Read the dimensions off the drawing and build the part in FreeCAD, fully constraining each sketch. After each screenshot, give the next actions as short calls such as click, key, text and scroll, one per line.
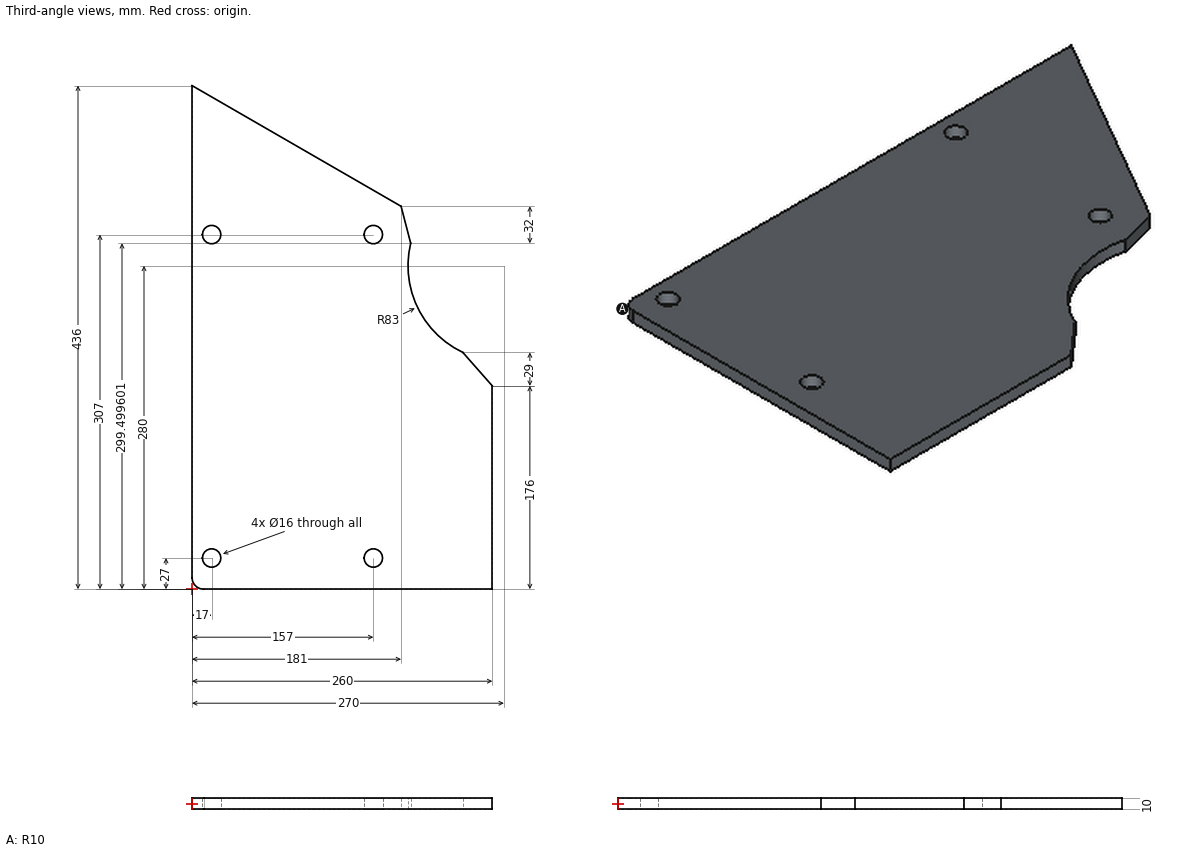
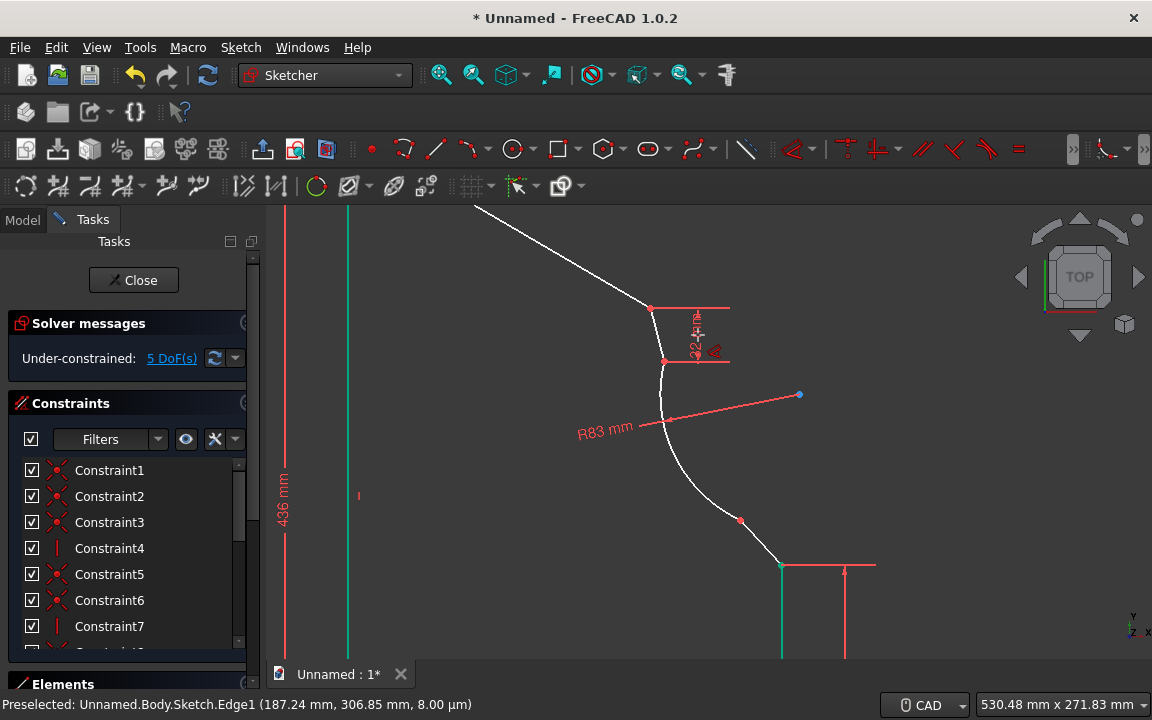
click(769, 552)
click(816, 543)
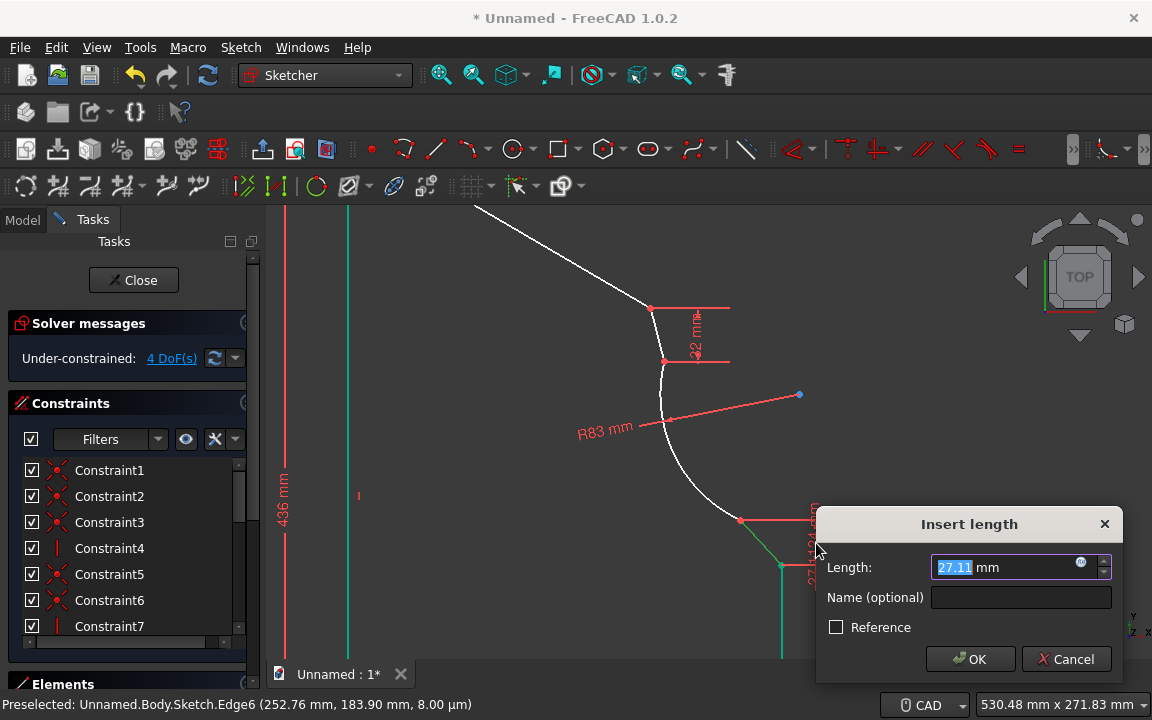
text(29)
key(Return)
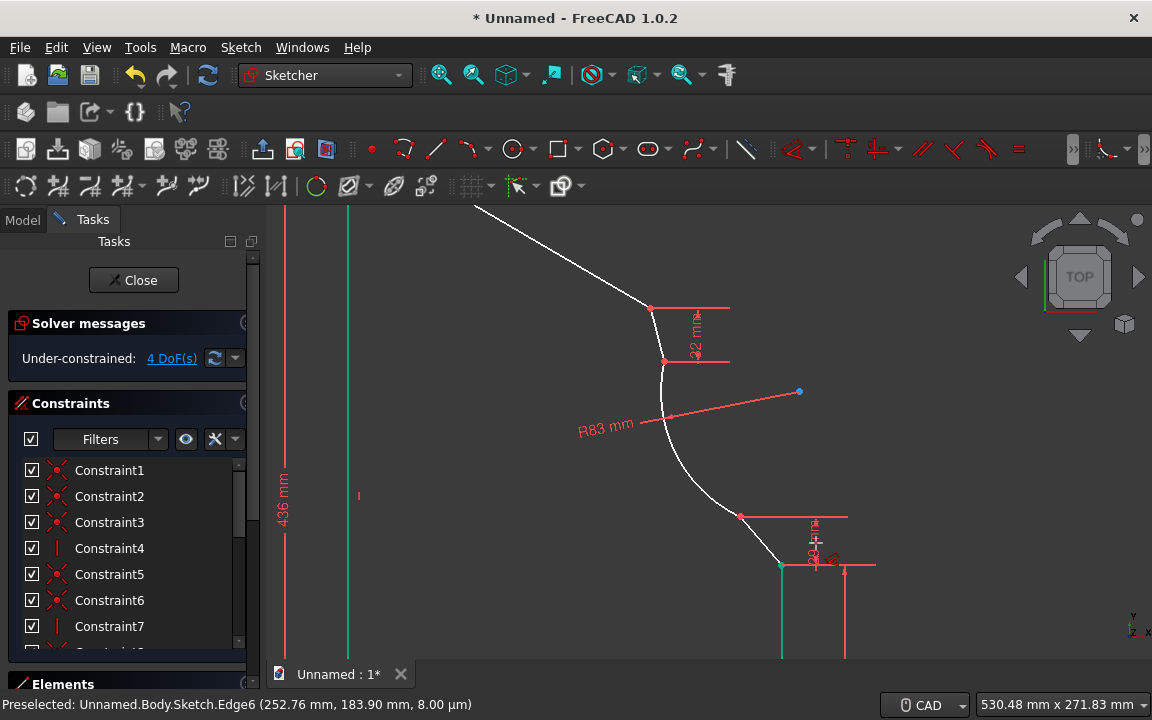
click(651, 308)
click(499, 274)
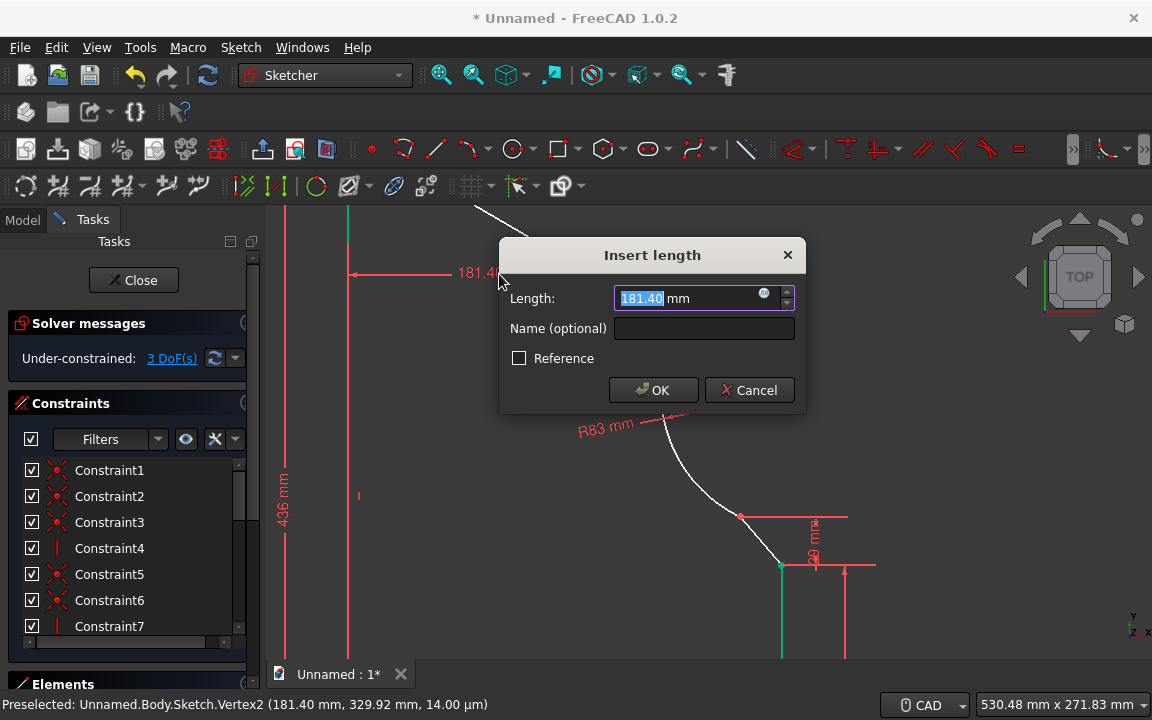
text(181)
key(Return)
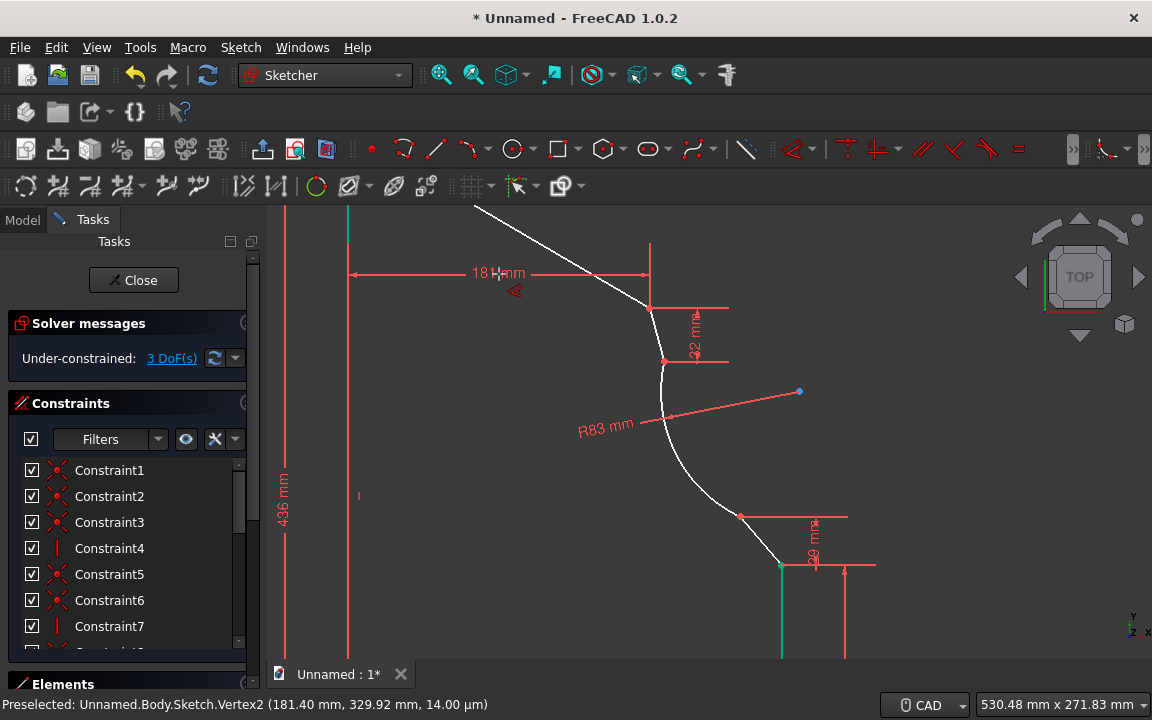
click(800, 392)
click(574, 358)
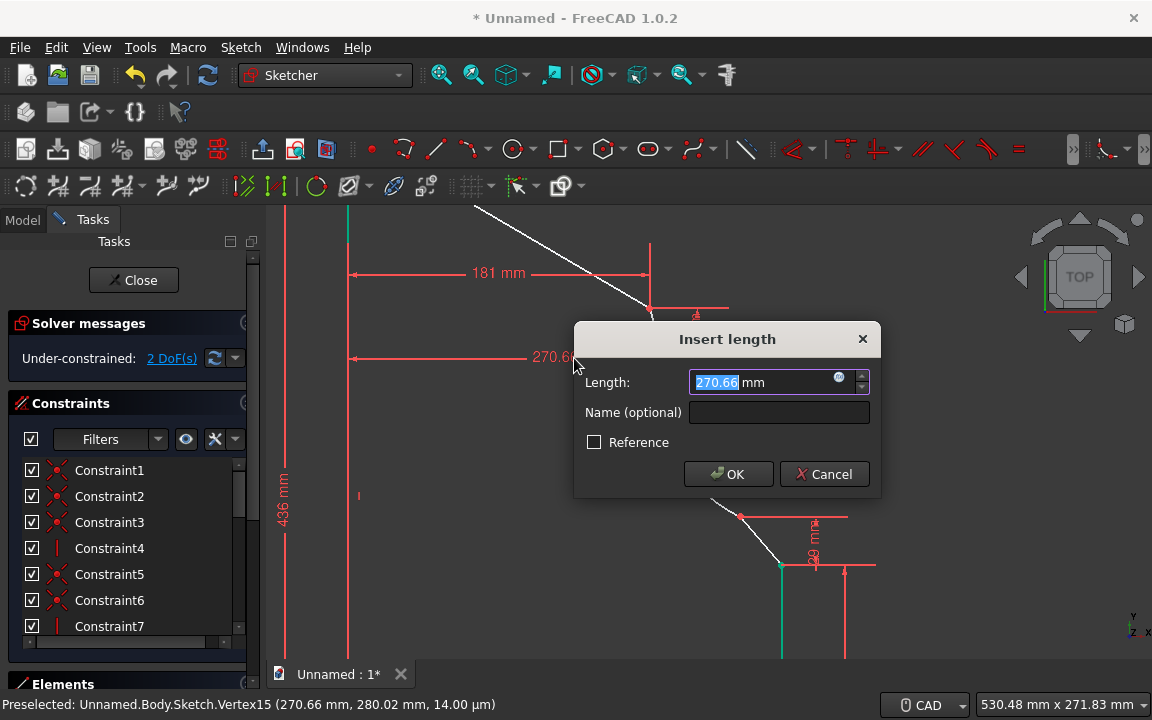
text(270)
key(Return)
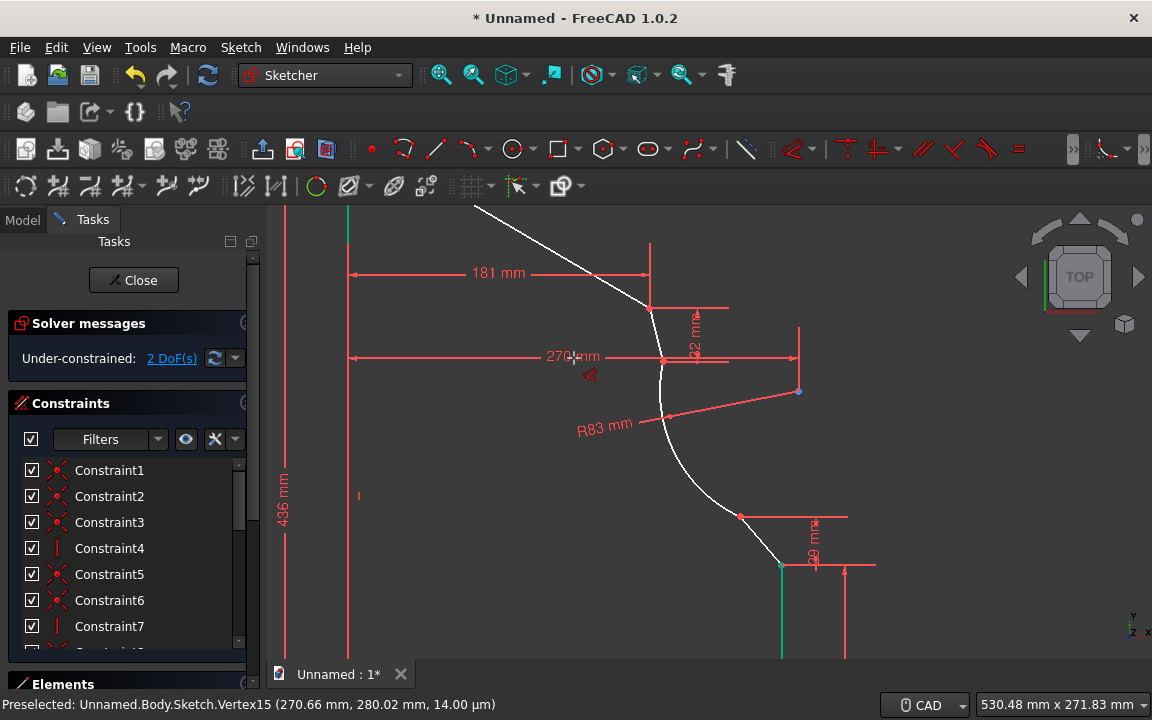
click(799, 391)
click(833, 511)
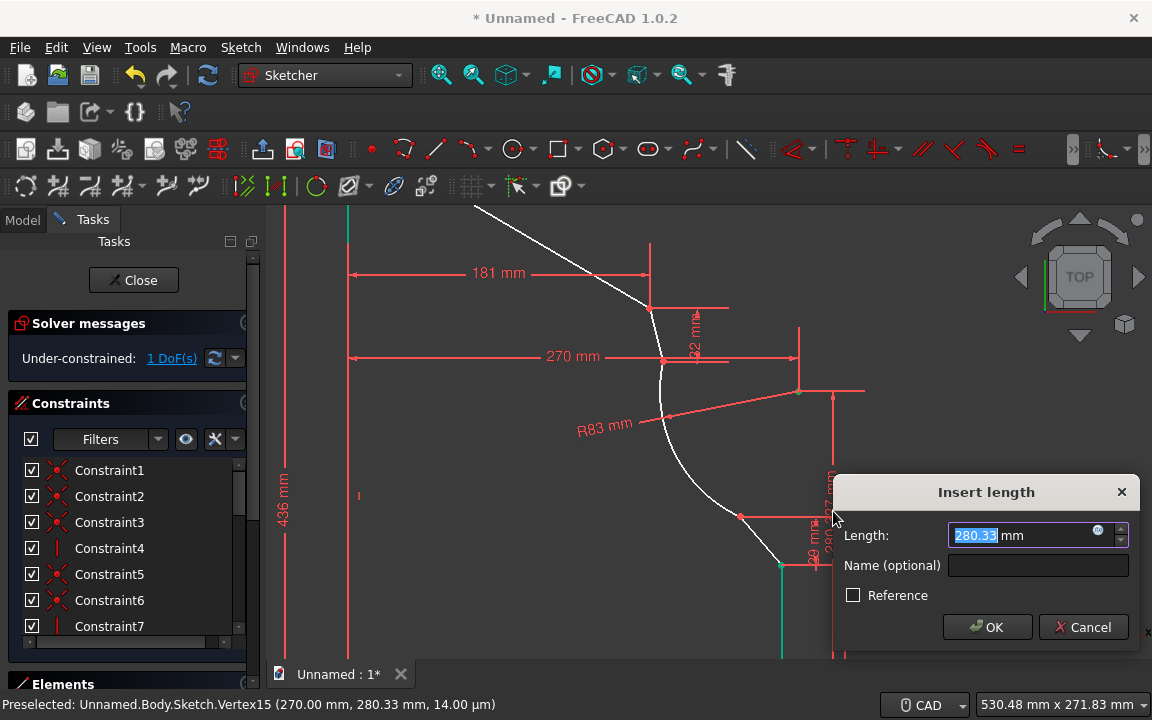
text(280)
key(Return)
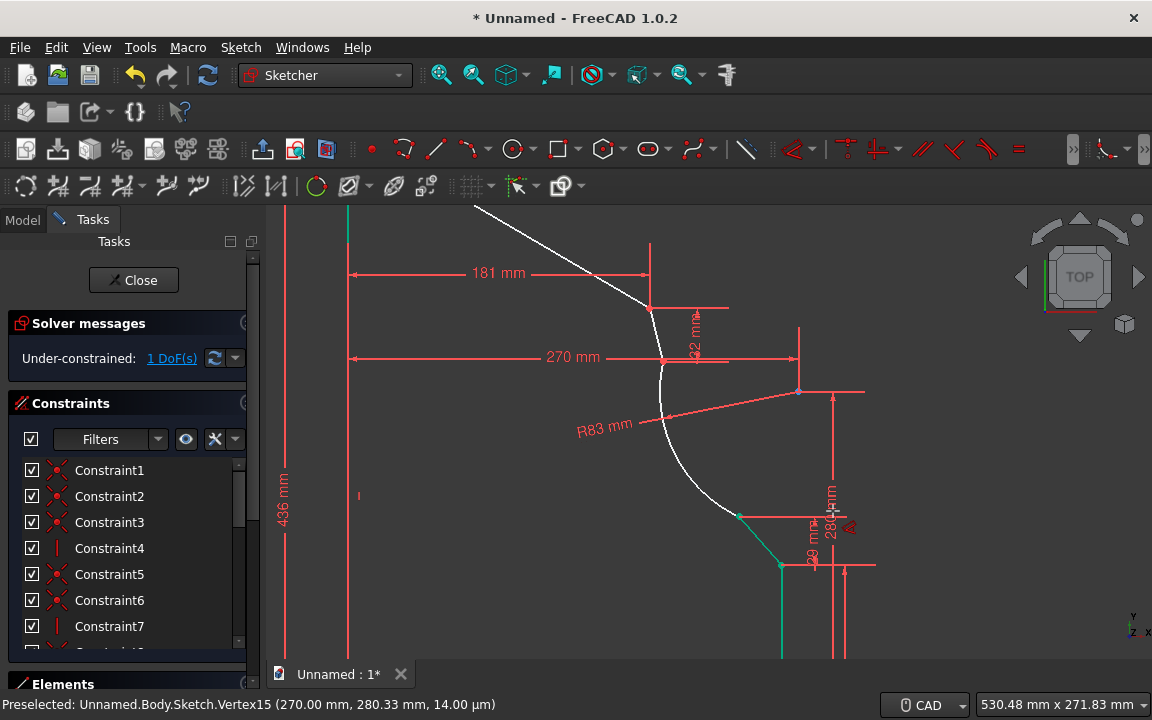
click(663, 362)
click(314, 434)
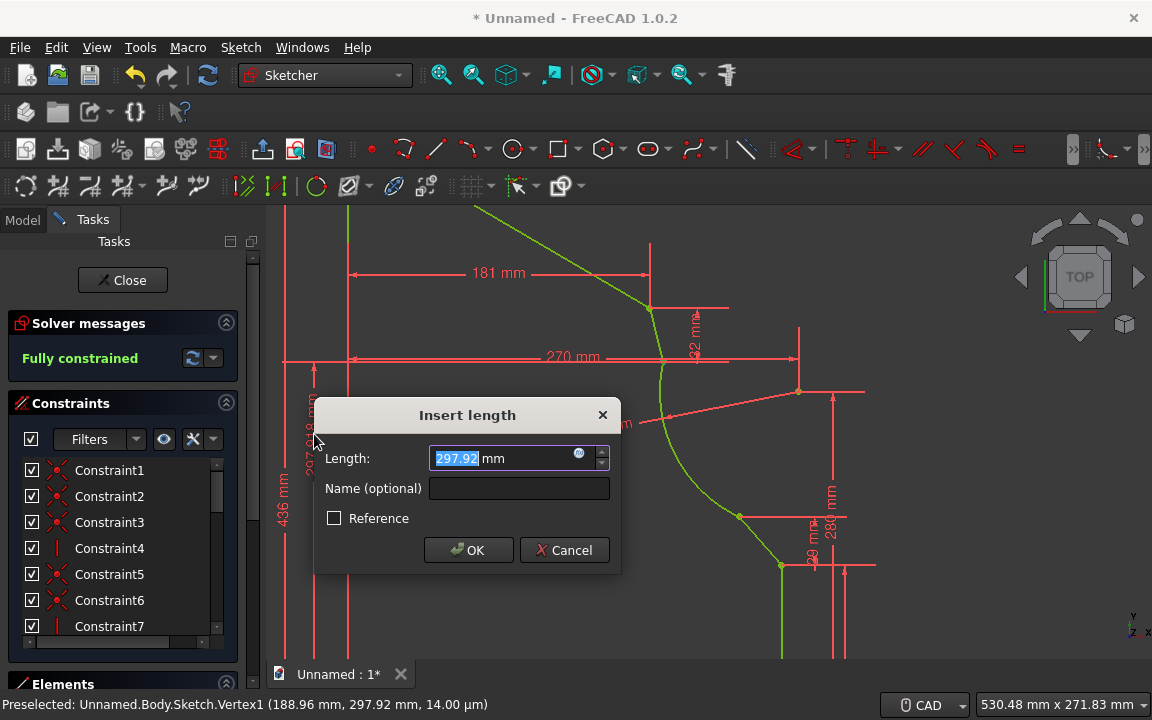
text(299.499601)
key(Return)
key(Escape)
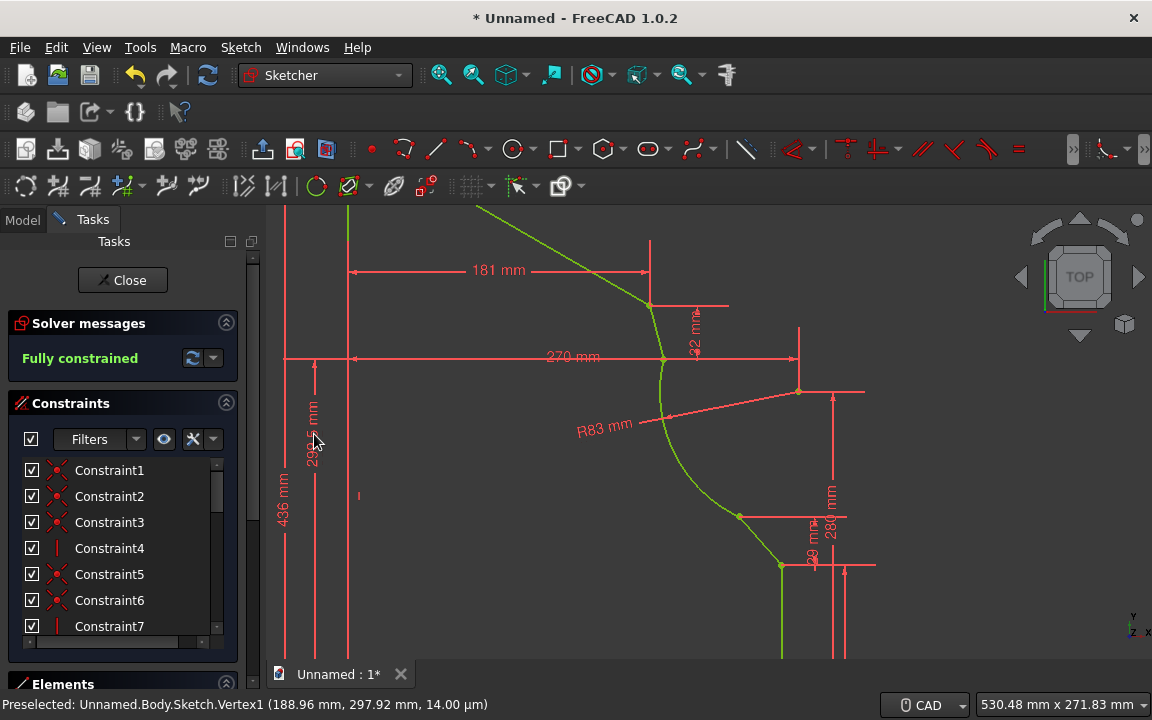
click(123, 280)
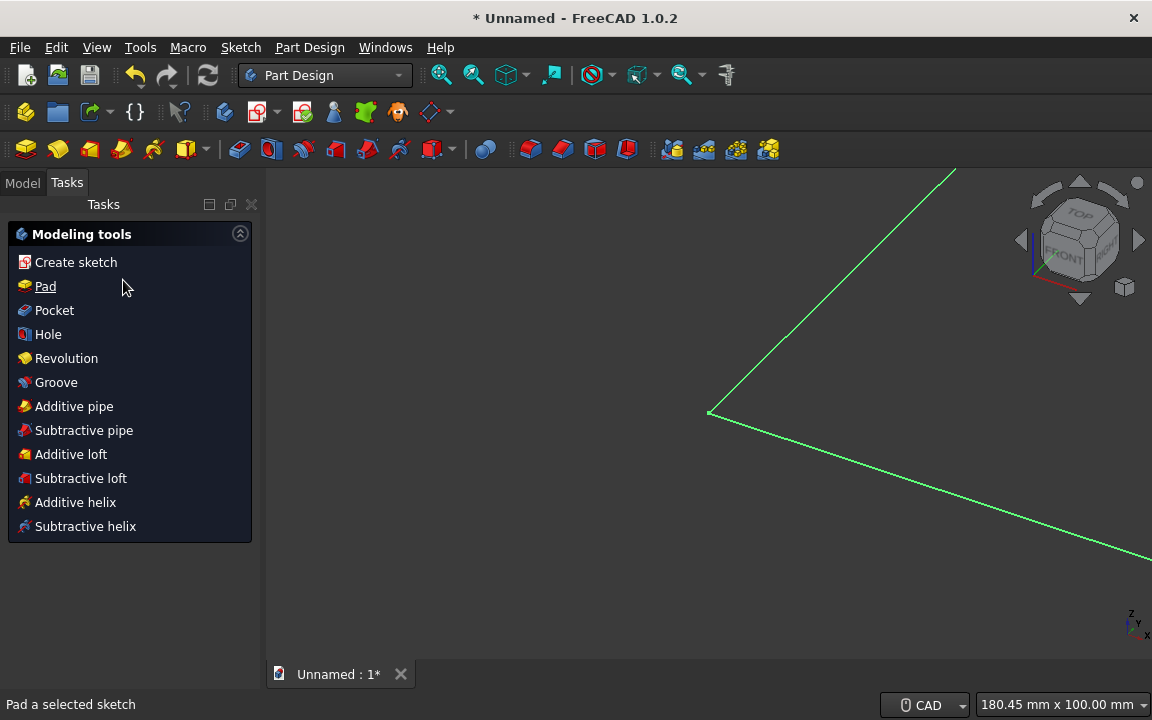
click(26, 150)